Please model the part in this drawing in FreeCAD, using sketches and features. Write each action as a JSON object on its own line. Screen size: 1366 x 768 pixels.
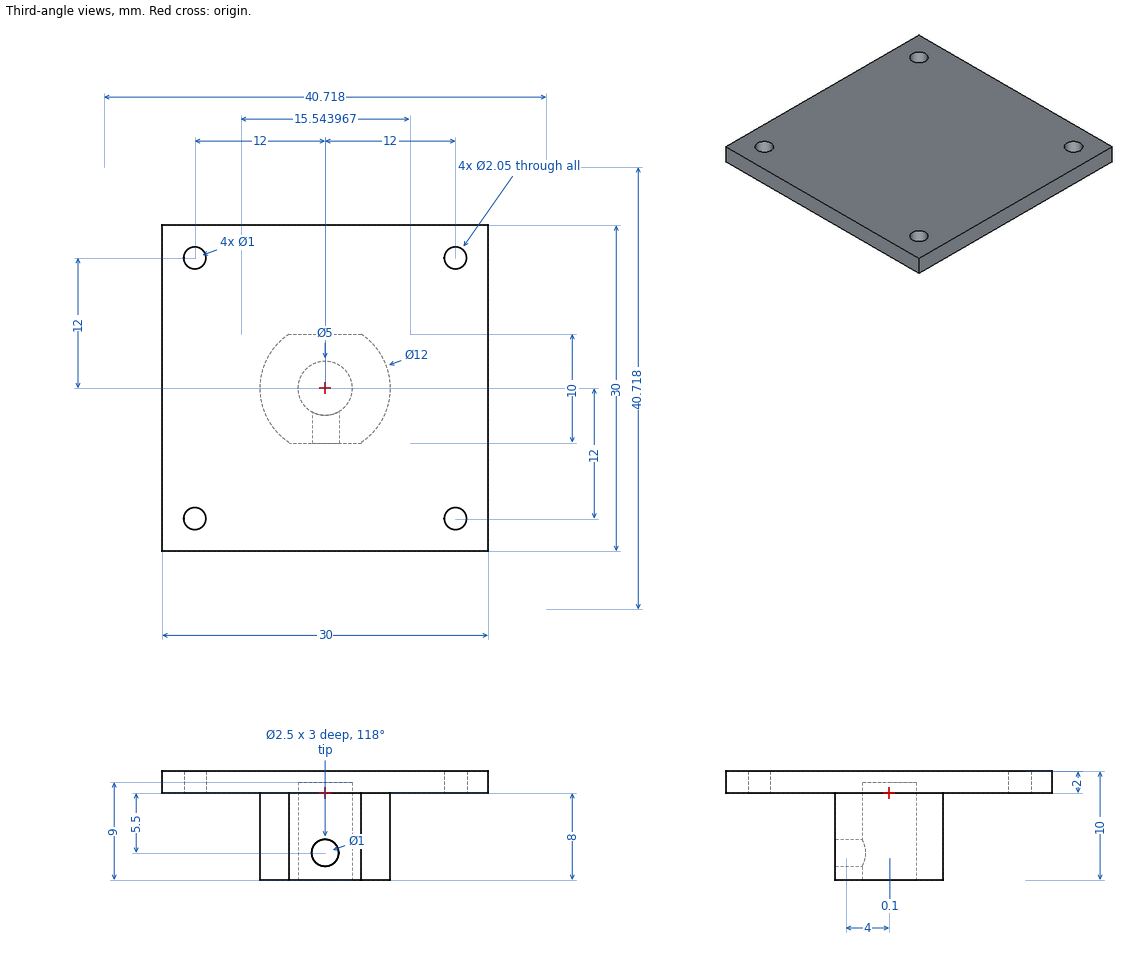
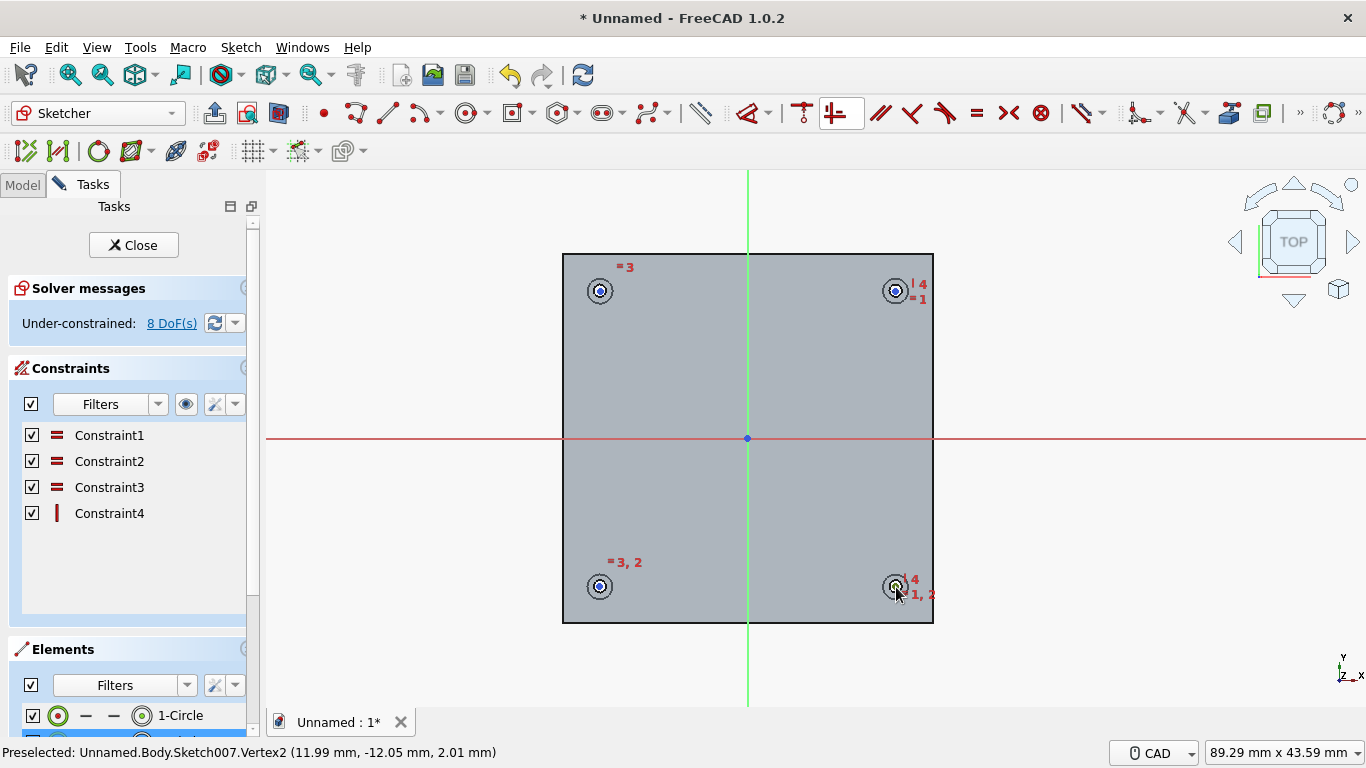
{"action": "left_click", "coordinate": [600, 587]}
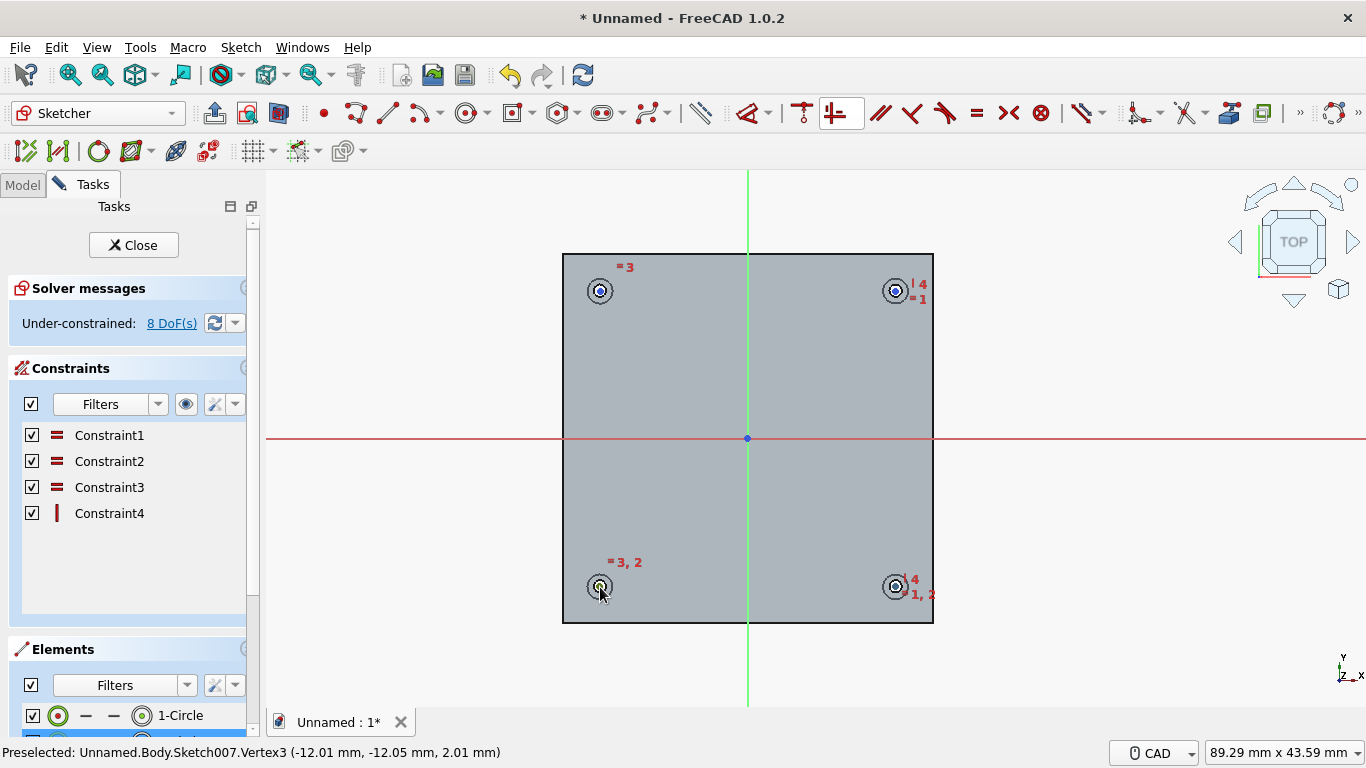
{"action": "key", "text": "h"}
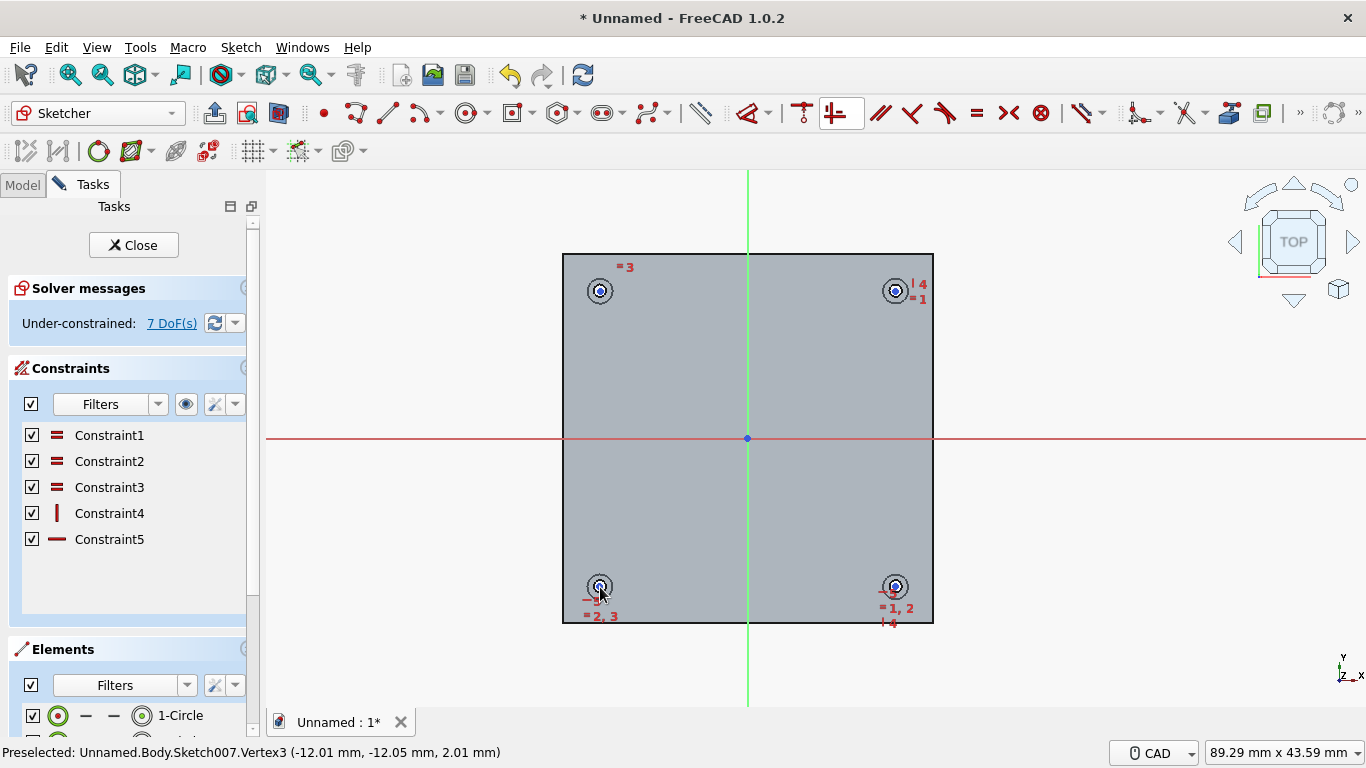
{"action": "left_click", "coordinate": [600, 587]}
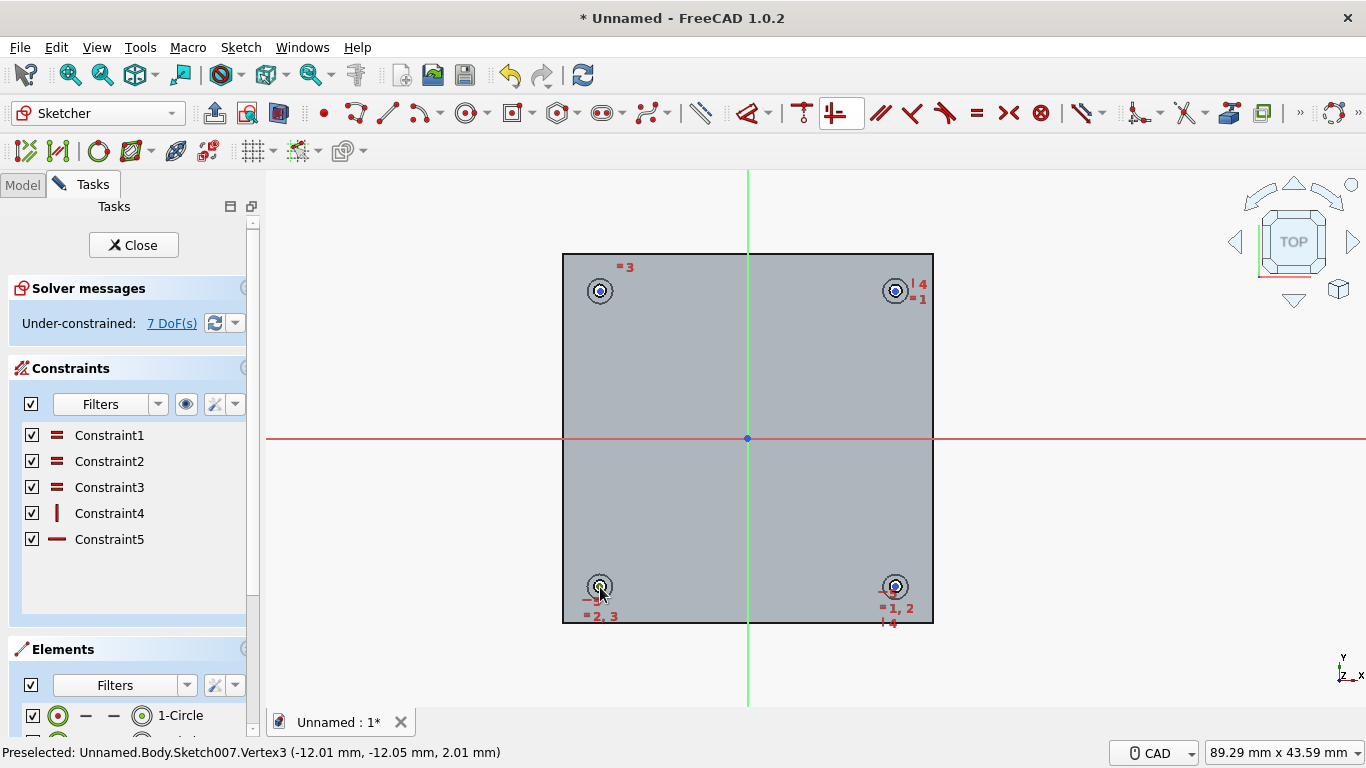
{"action": "left_click", "coordinate": [600, 291]}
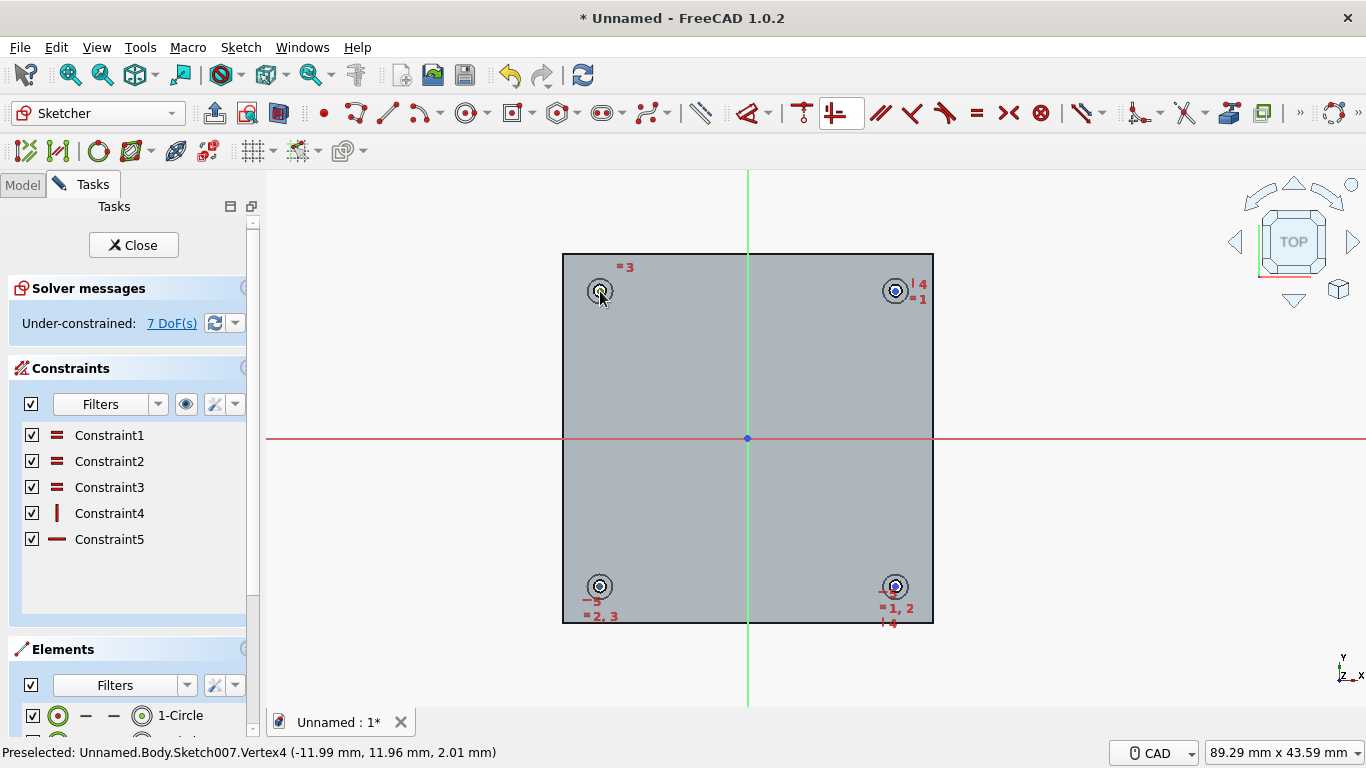
{"action": "key", "text": "v"}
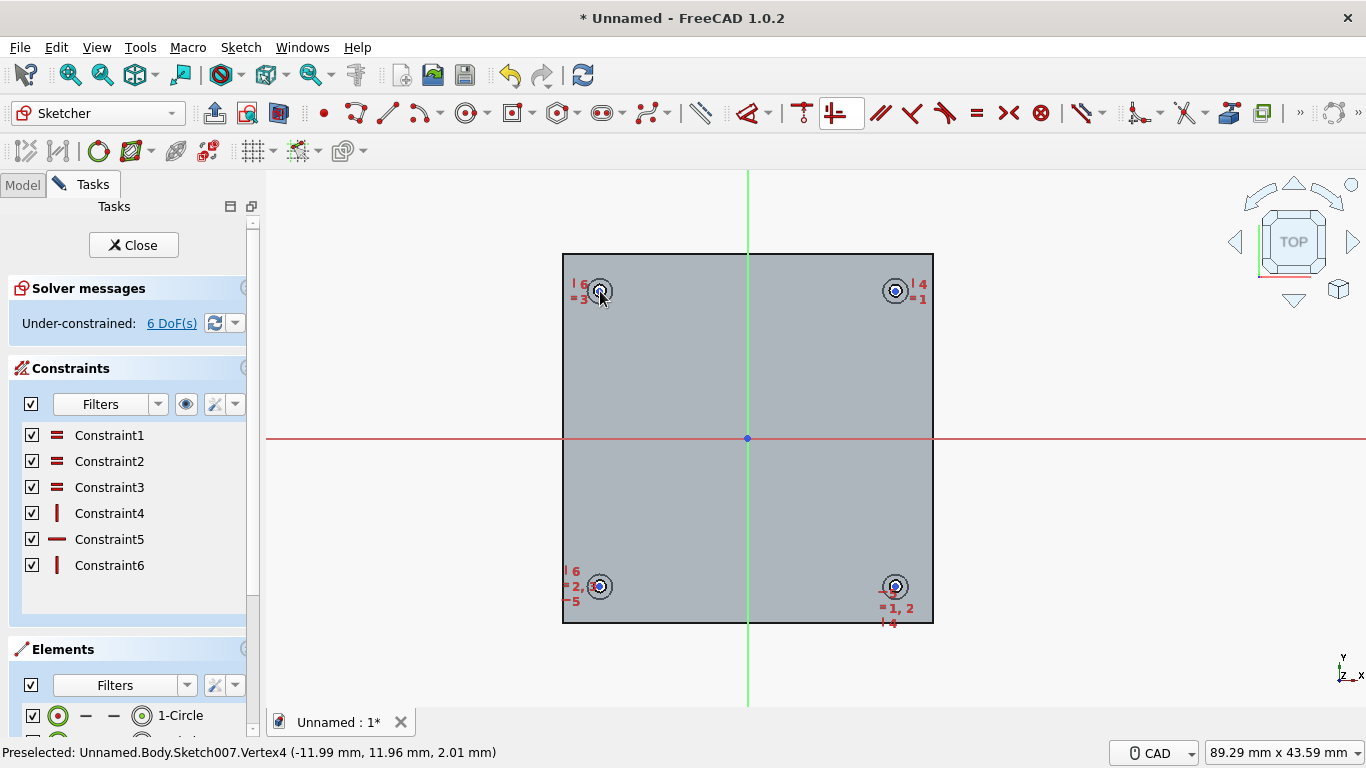
{"action": "left_click", "coordinate": [896, 291]}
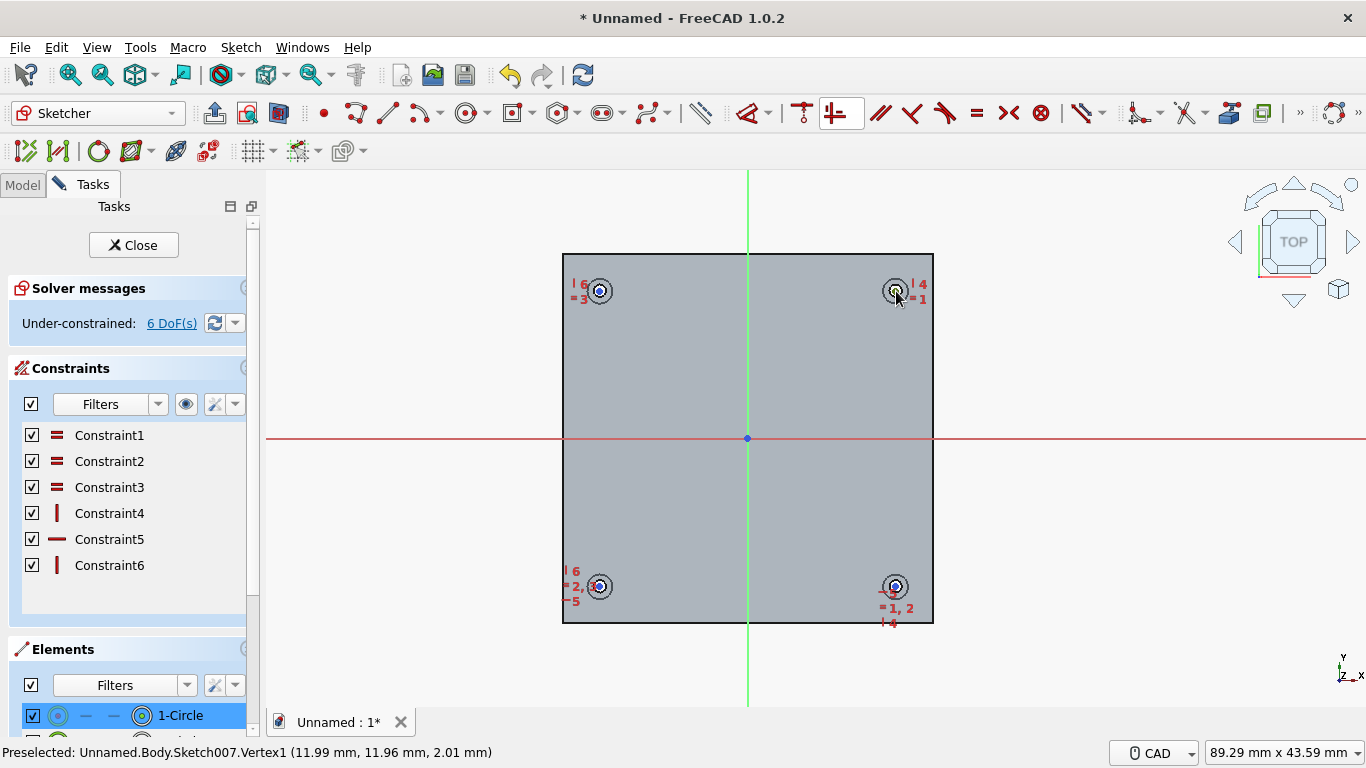
{"action": "left_click", "coordinate": [600, 291]}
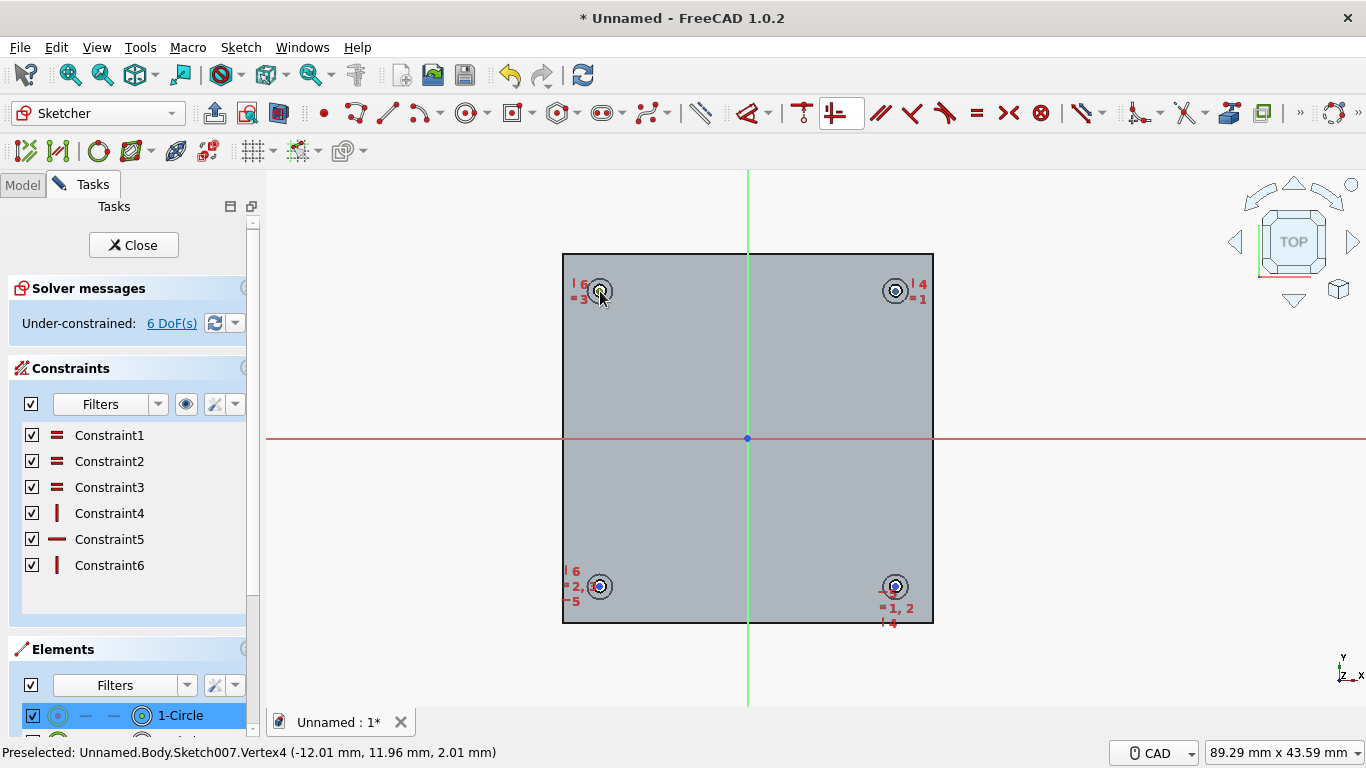
{"action": "key", "text": "h"}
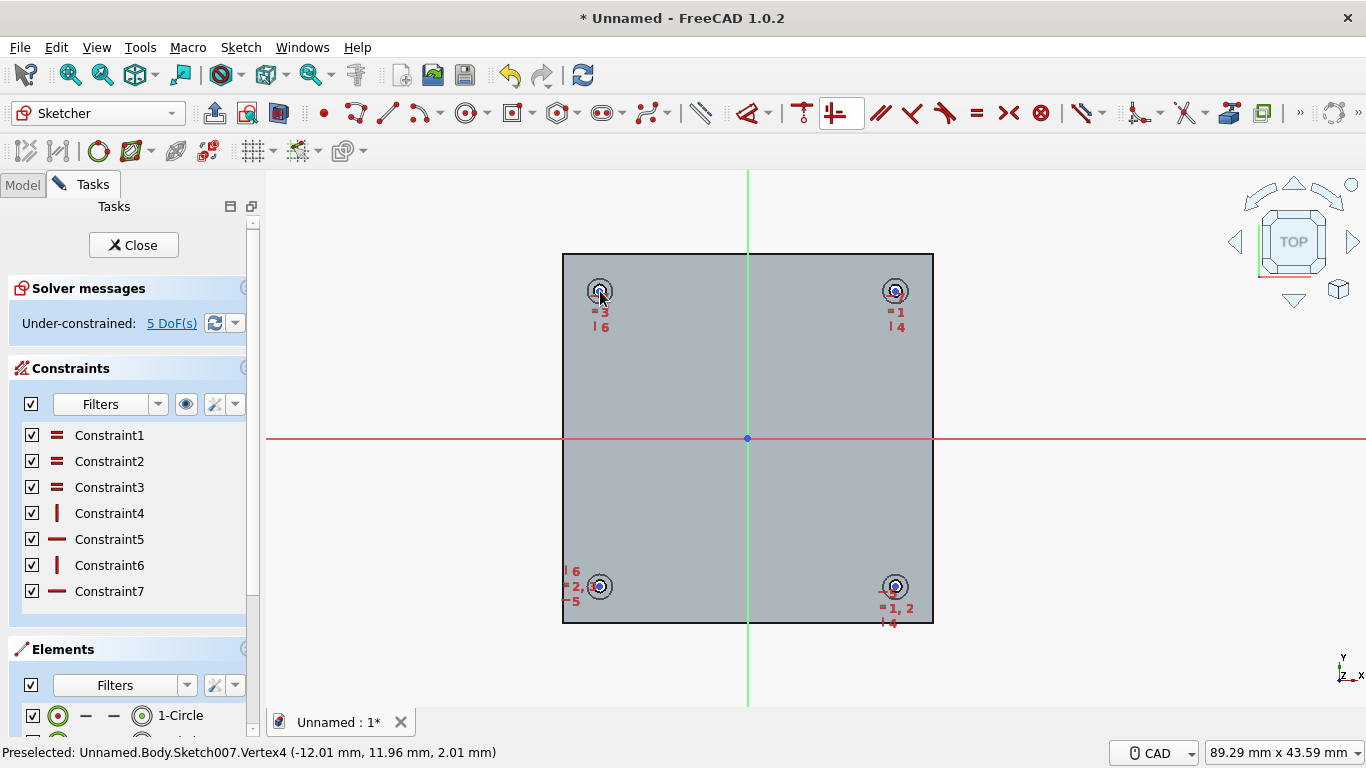
{"action": "key", "text": "d"}